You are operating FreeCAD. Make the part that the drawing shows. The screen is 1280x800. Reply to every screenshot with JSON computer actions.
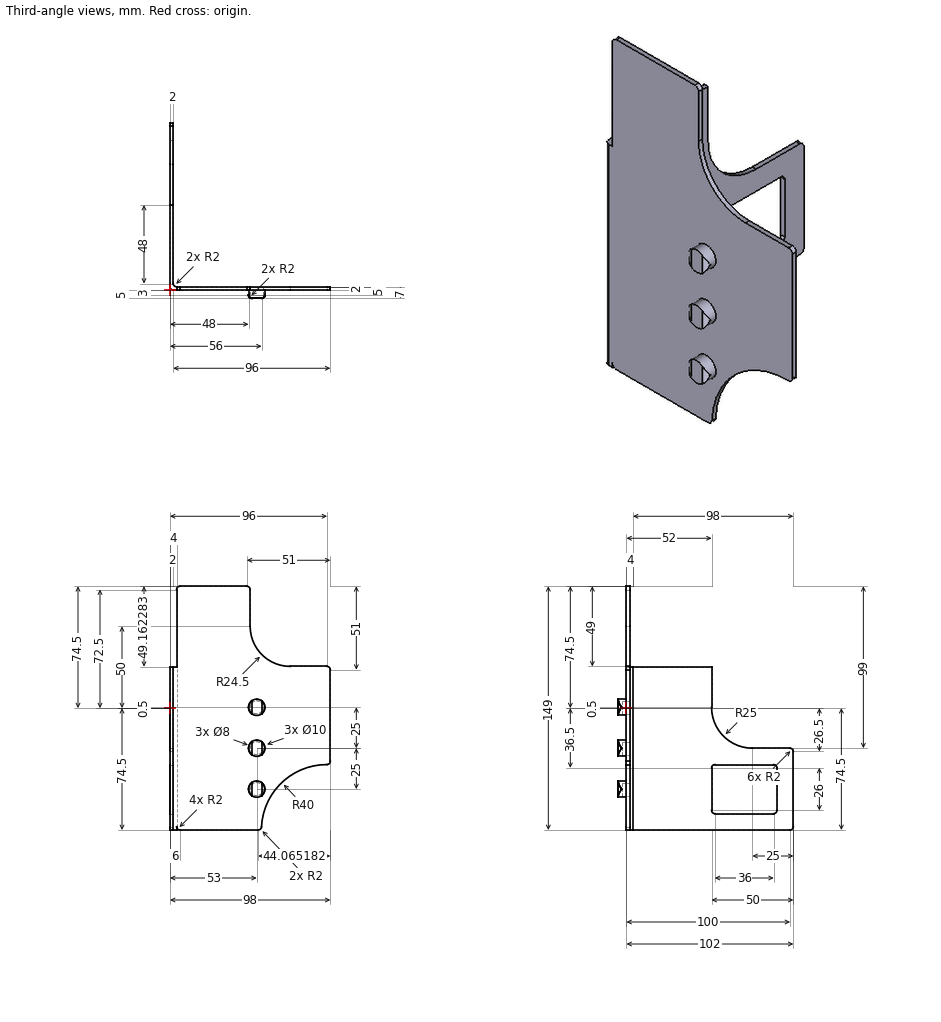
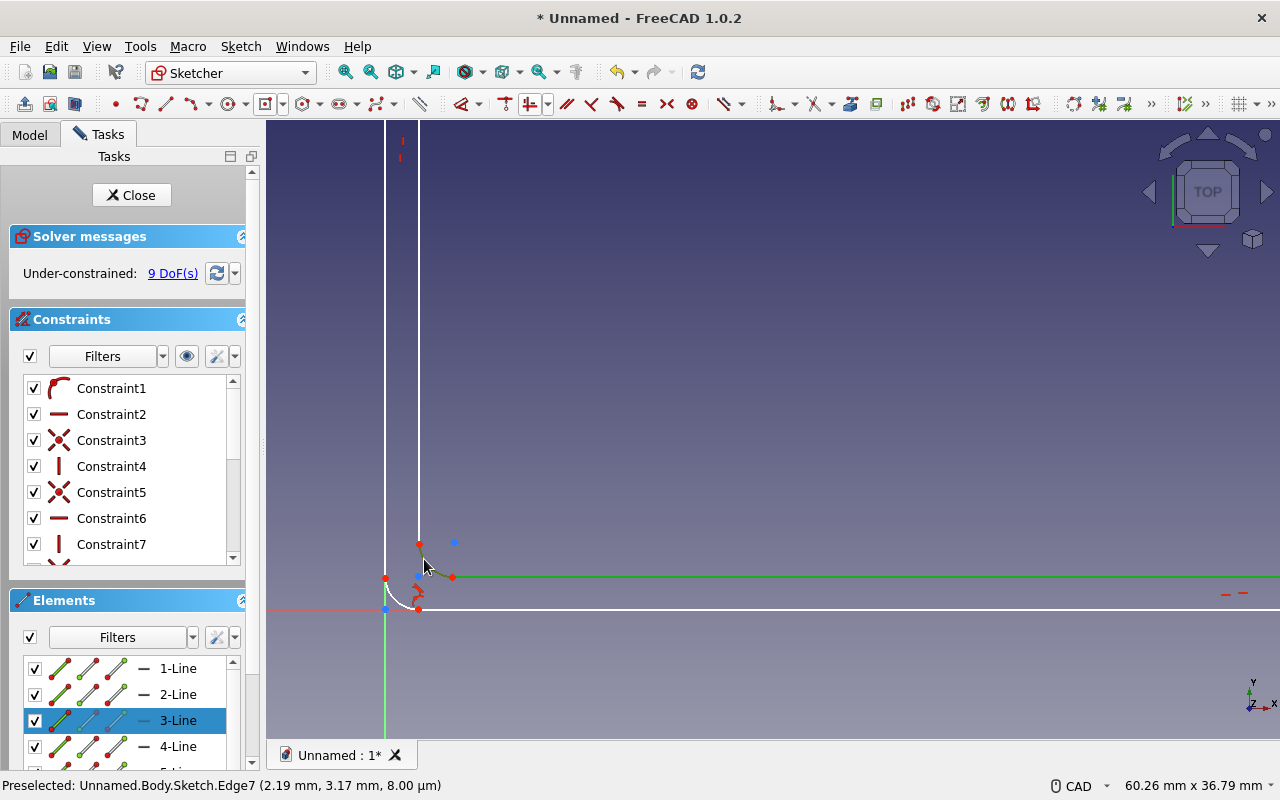
{"action": "key", "text": "t"}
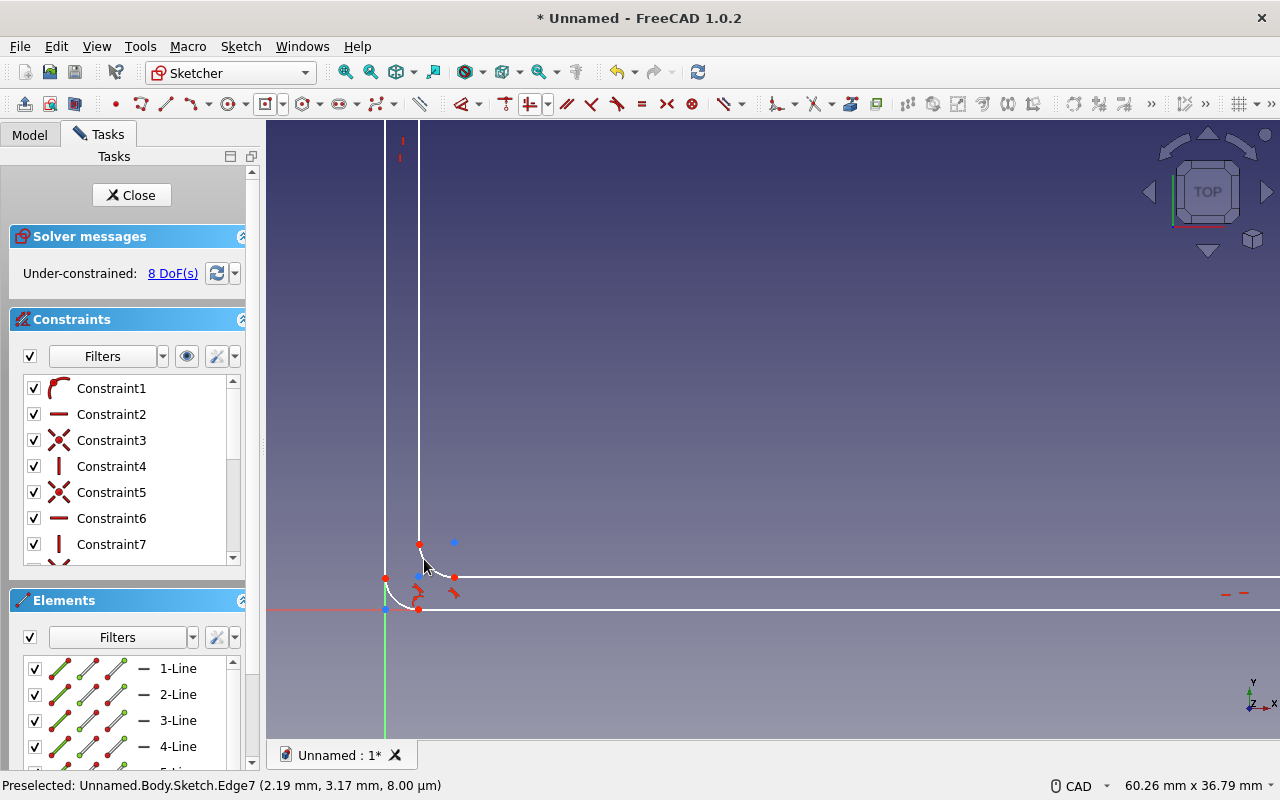
{"action": "left_click", "coordinate": [419, 302]}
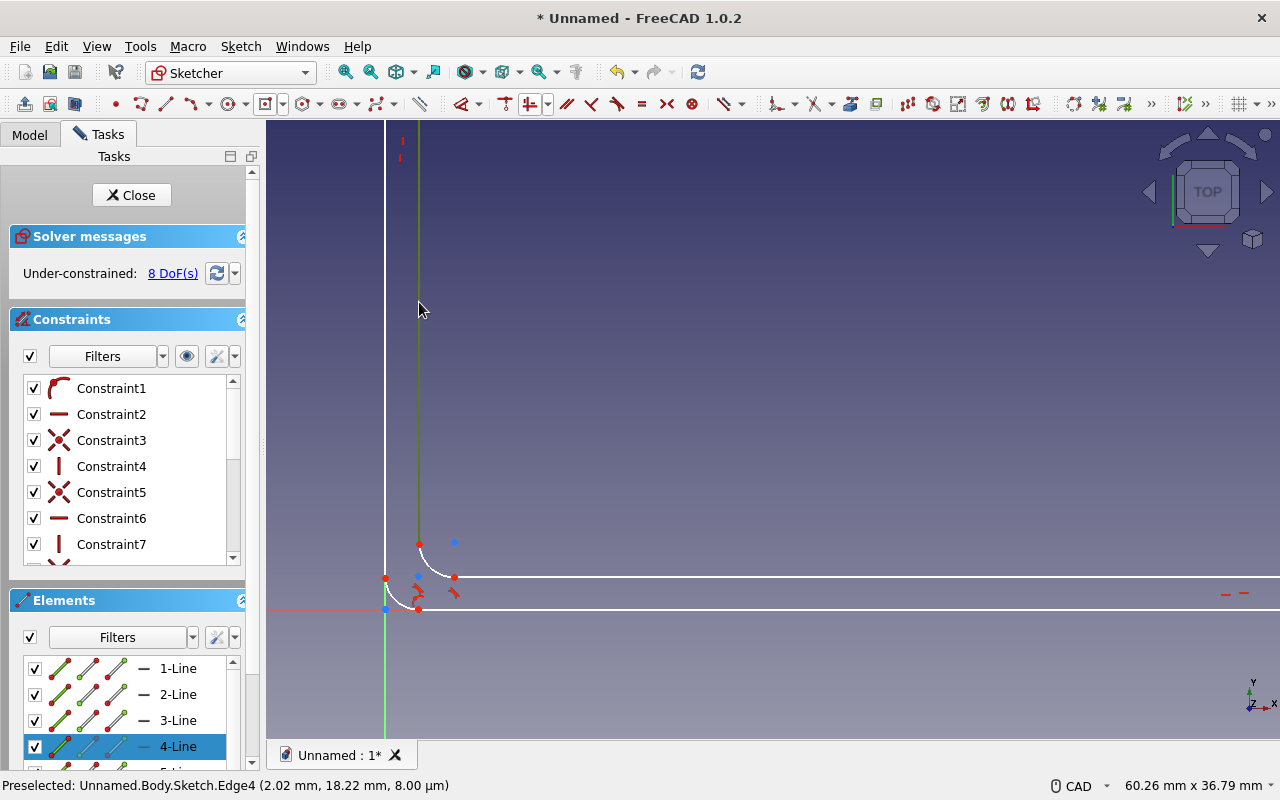
{"action": "left_click", "coordinate": [424, 560]}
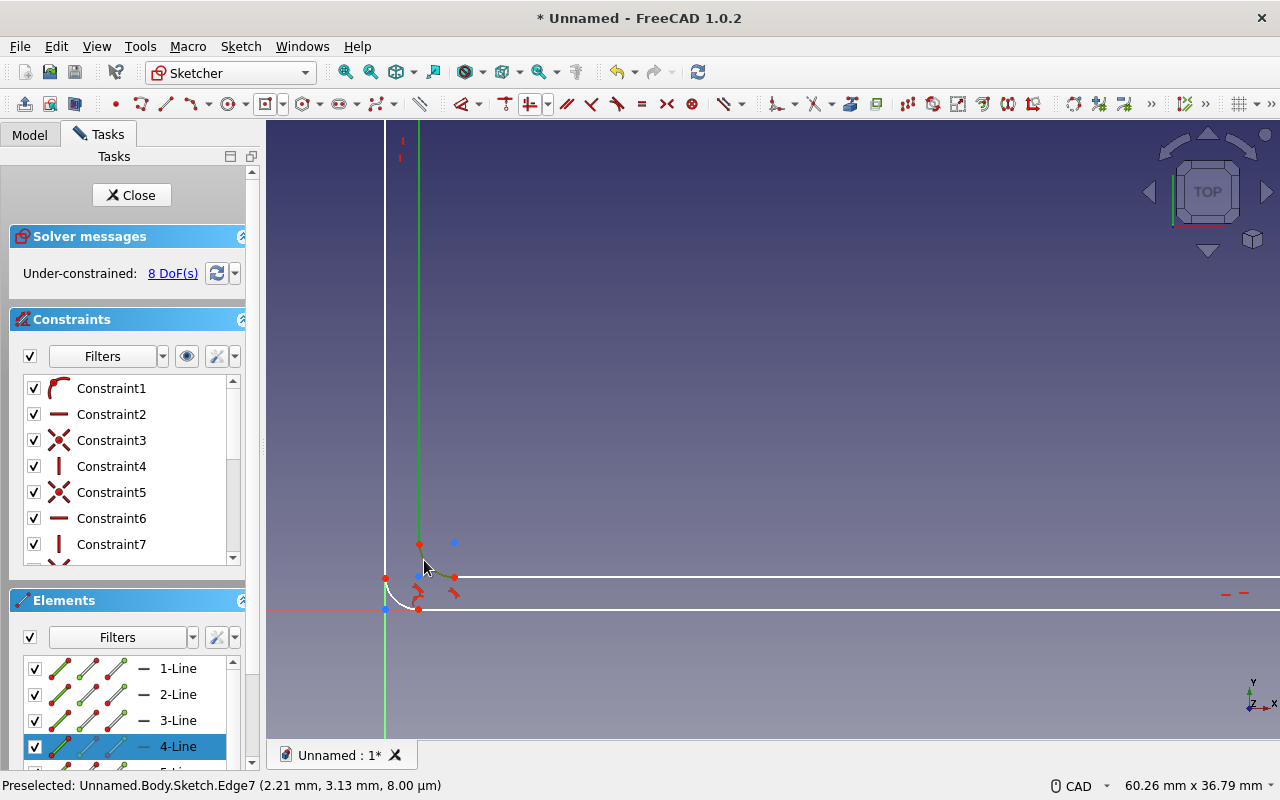
{"action": "key", "text": "t"}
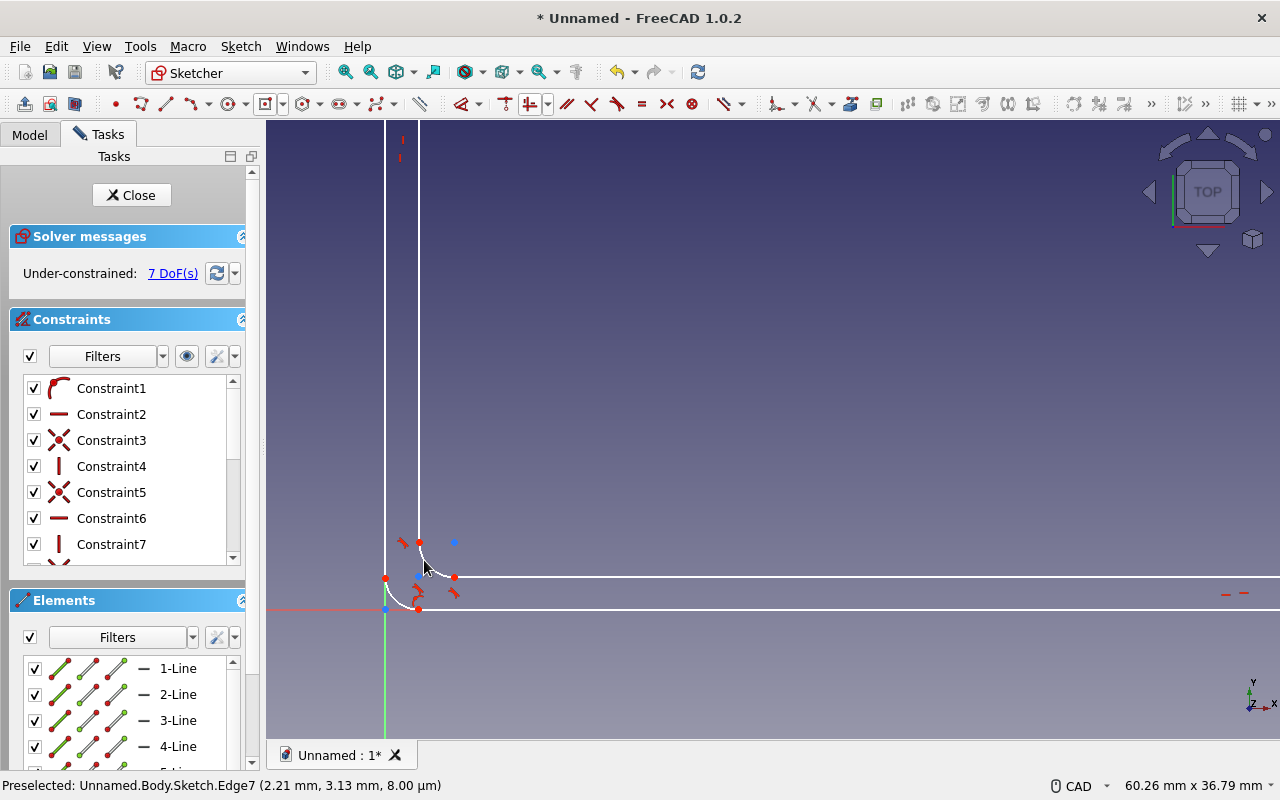
{"action": "left_click", "coordinate": [385, 326]}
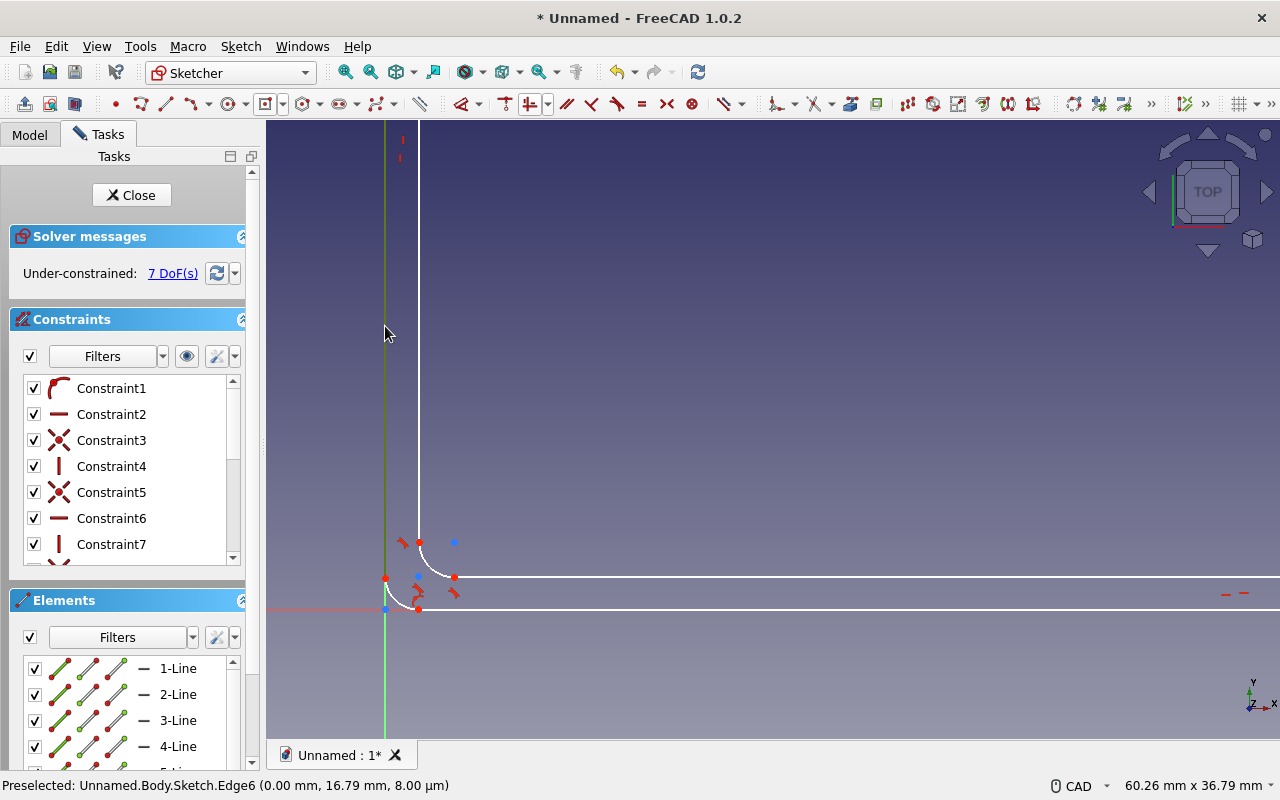
{"action": "left_click", "coordinate": [404, 606]}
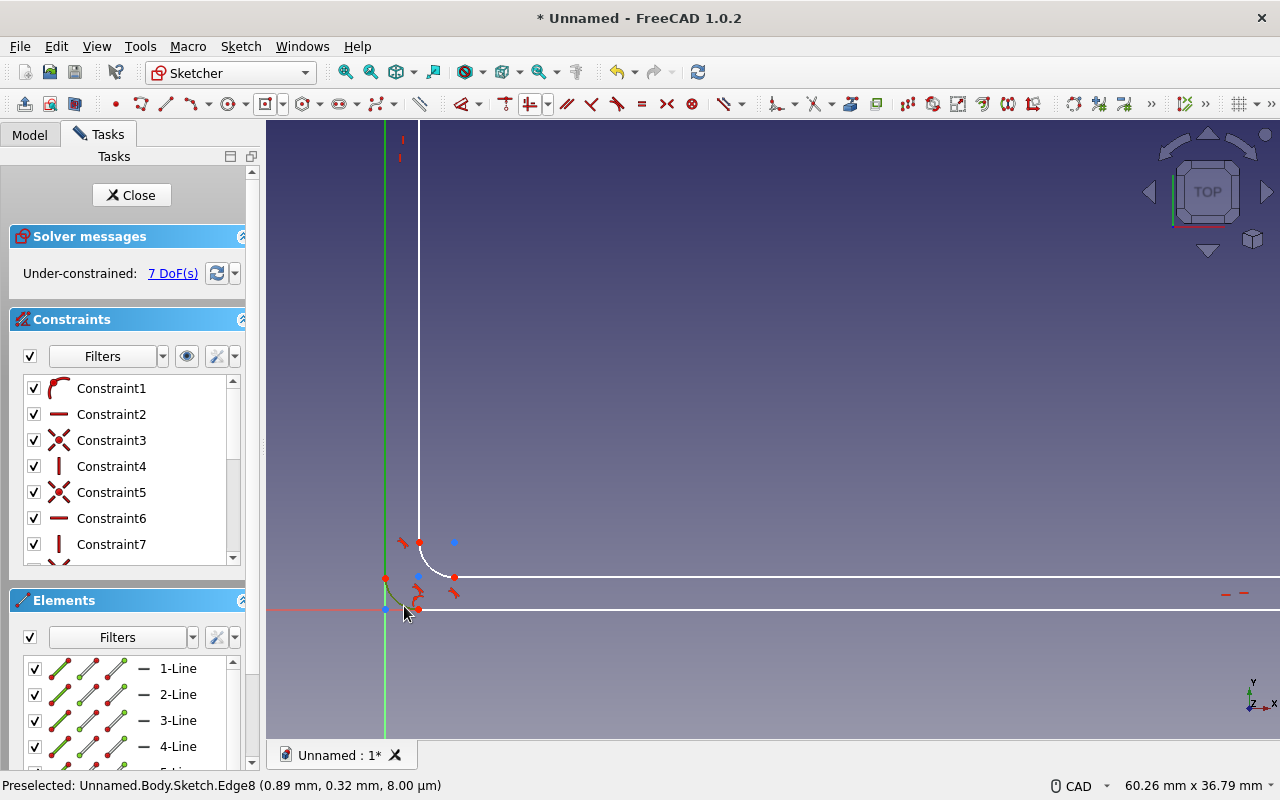
{"action": "key", "text": "t"}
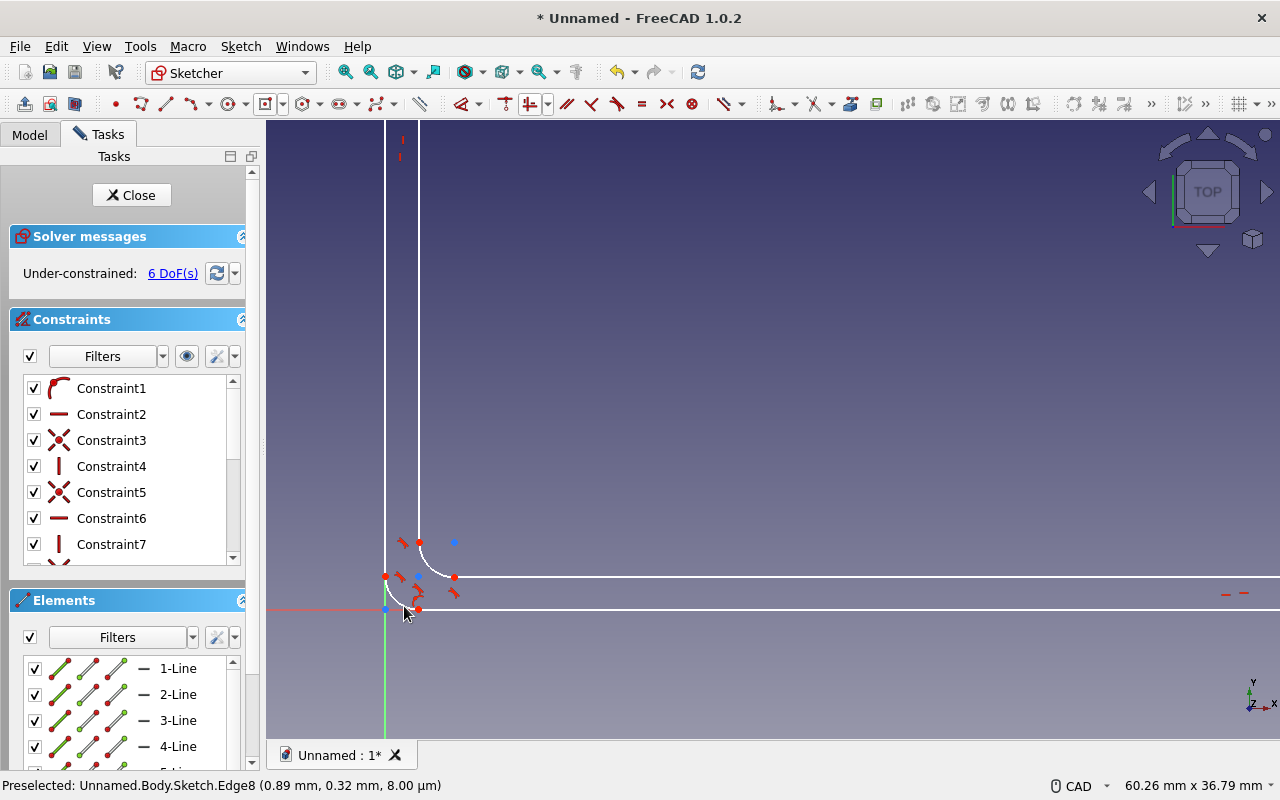
{"action": "left_click", "coordinate": [423, 558]}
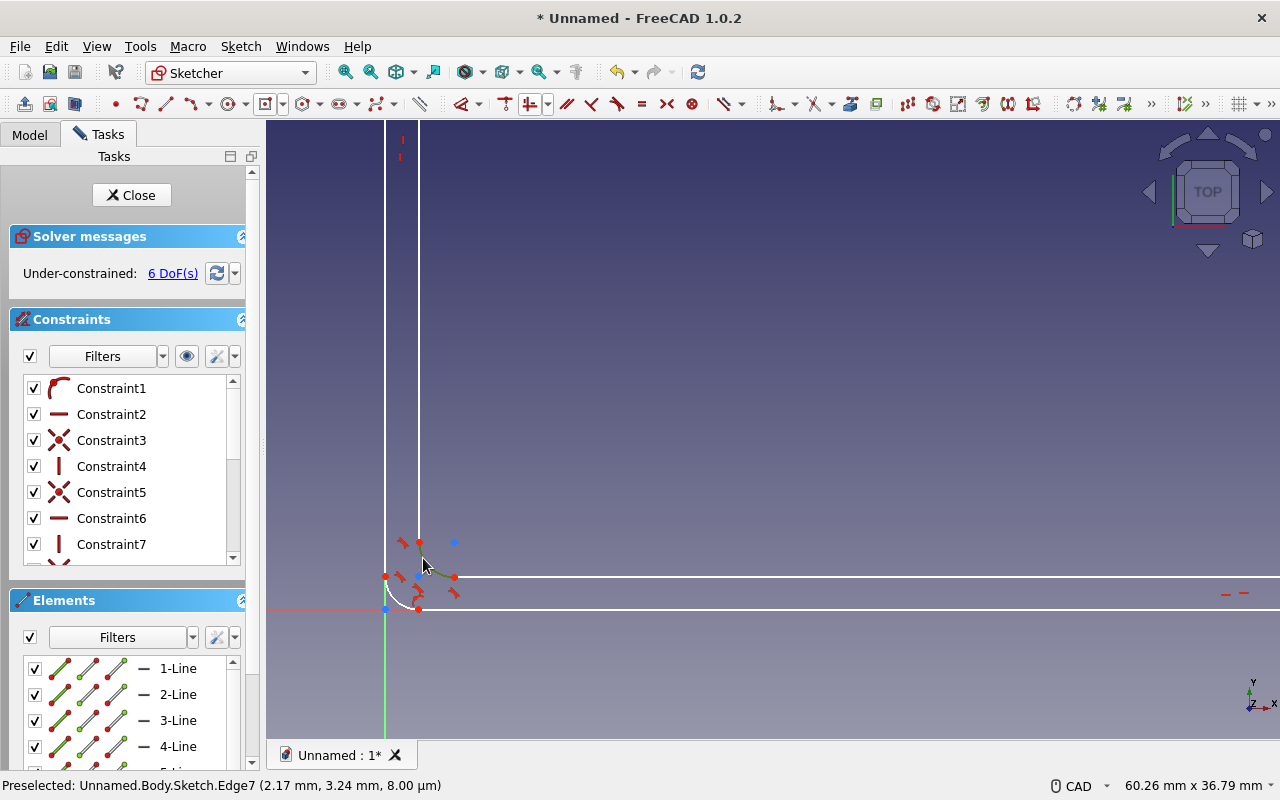
{"action": "left_click", "coordinate": [389, 592]}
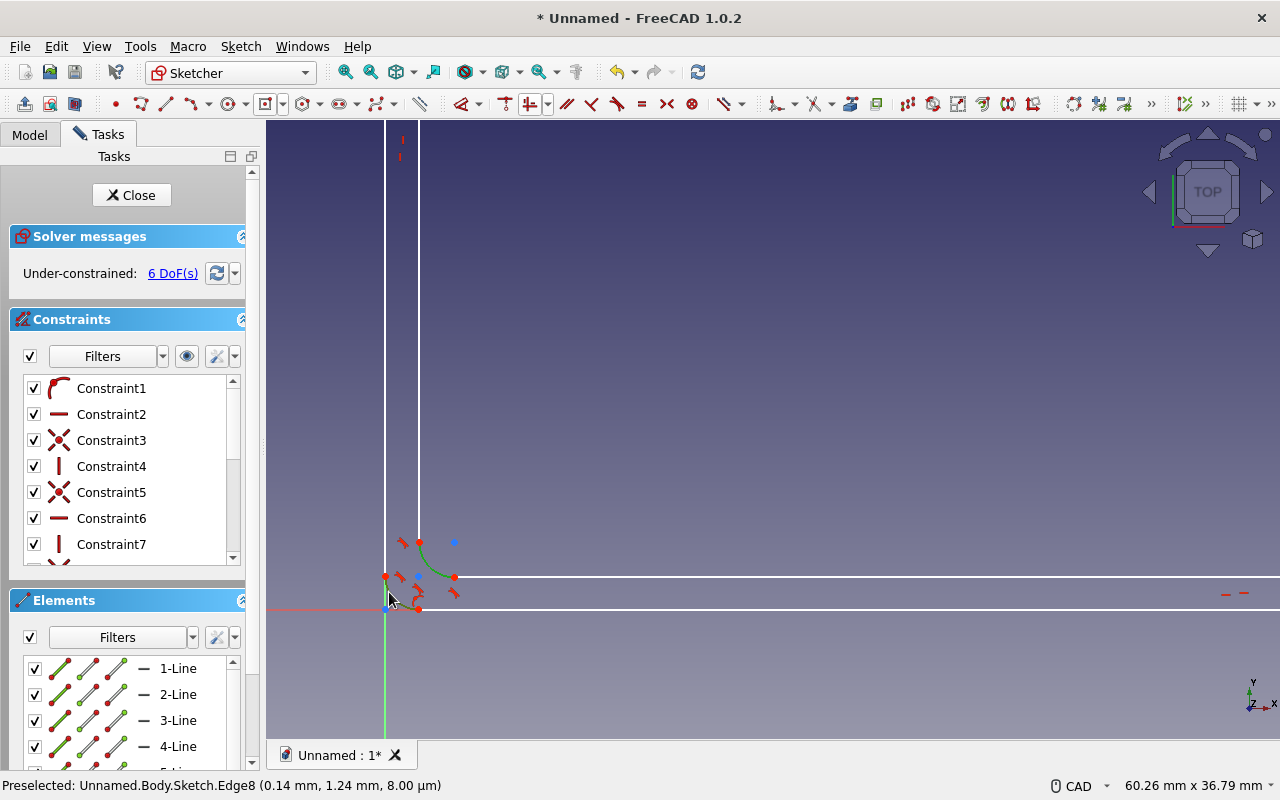
{"action": "key", "text": "e"}